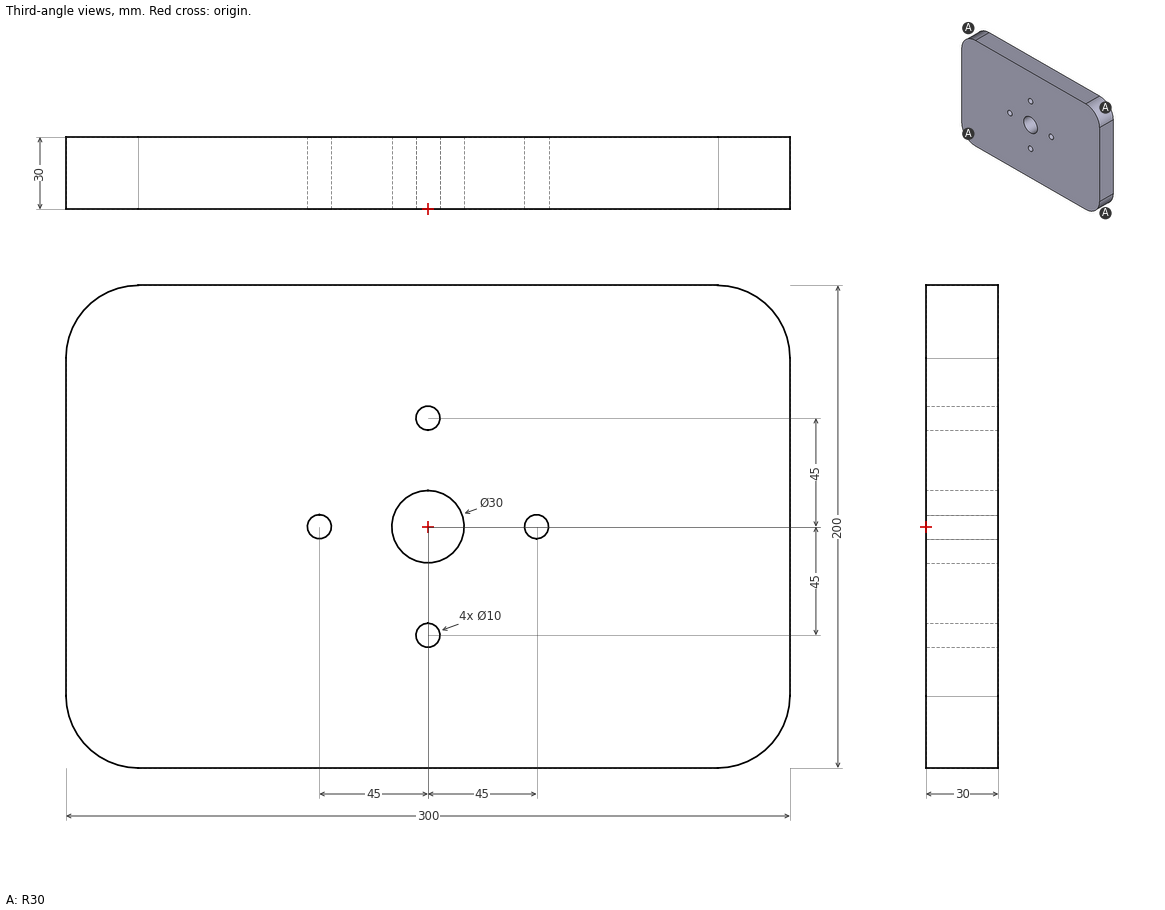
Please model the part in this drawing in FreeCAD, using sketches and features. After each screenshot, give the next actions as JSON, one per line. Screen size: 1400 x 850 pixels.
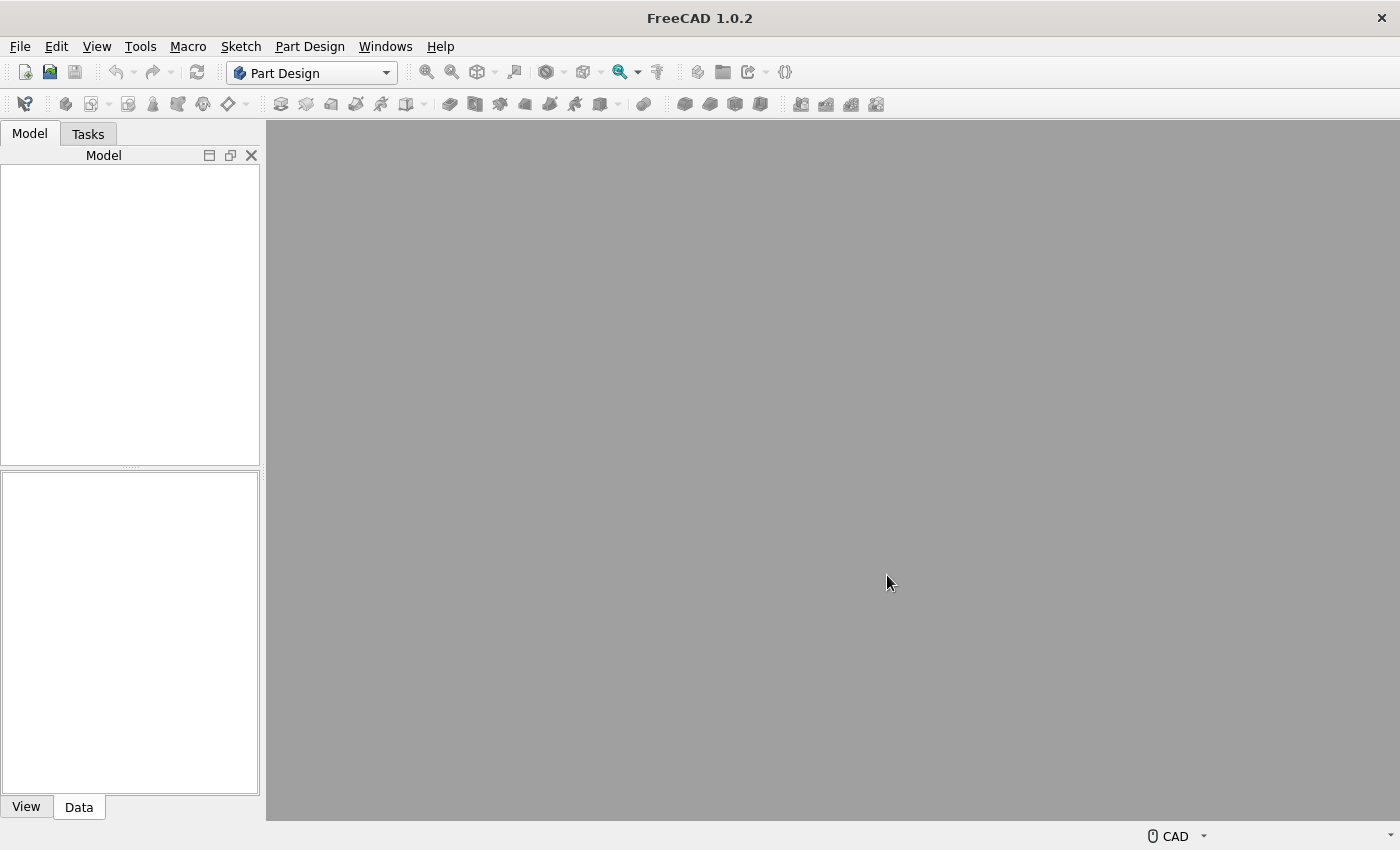
{"action": "key", "text": "ctrl+n"}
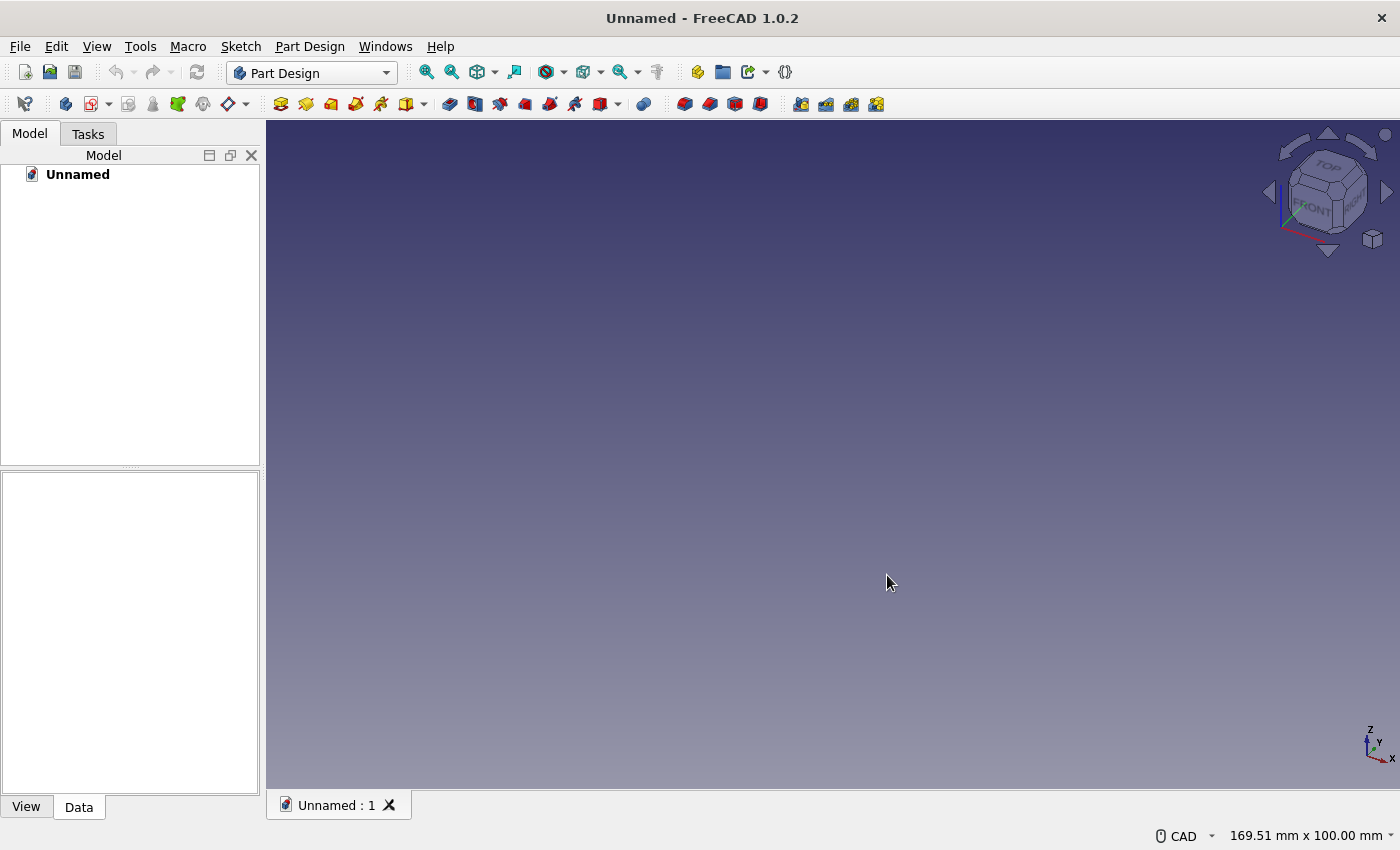
{"action": "left_click", "coordinate": [90, 104]}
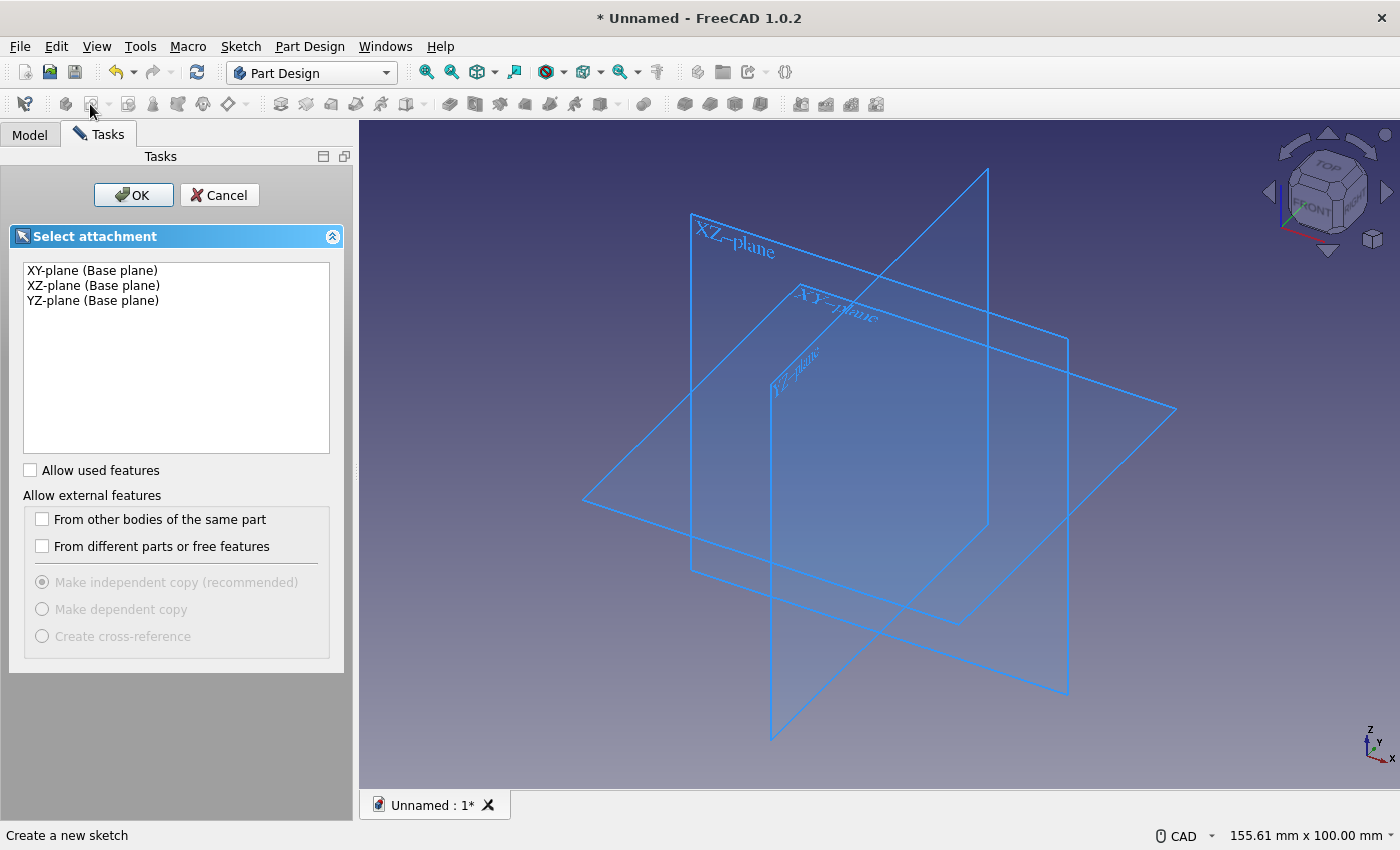
{"action": "left_click", "coordinate": [84, 286]}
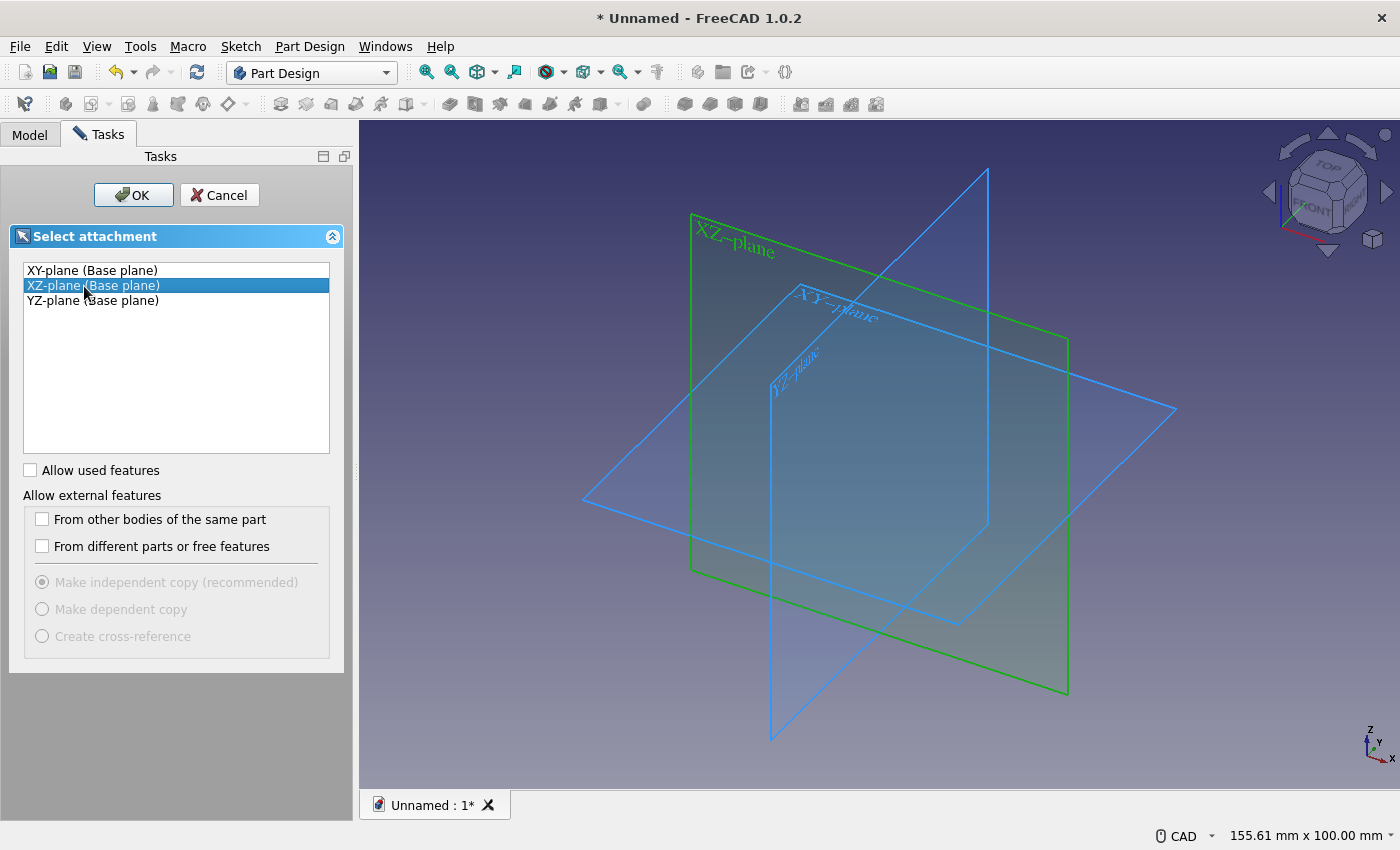
{"action": "left_click", "coordinate": [134, 195]}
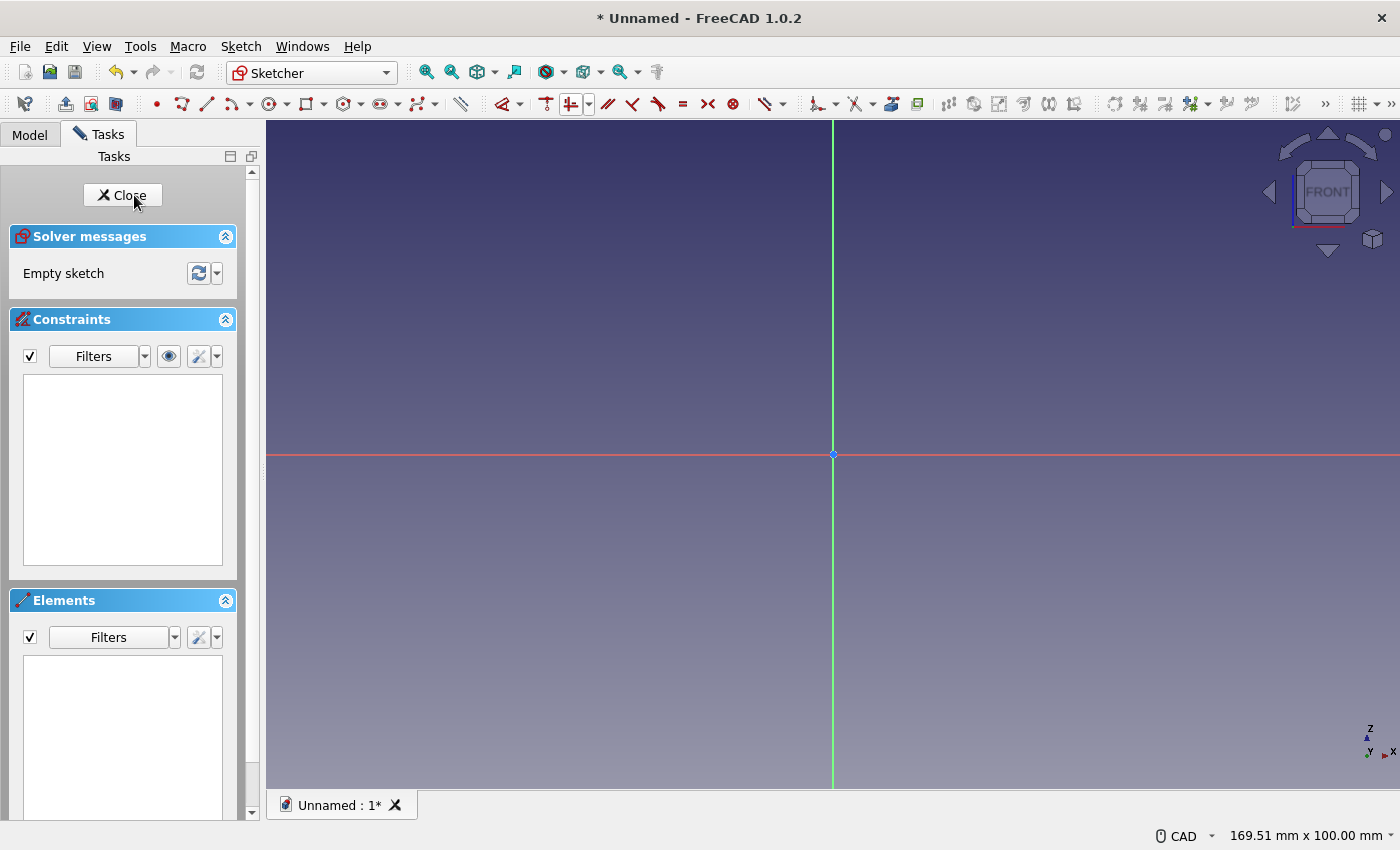
{"action": "scroll", "coordinate": [735, 454], "scroll_direction": "down", "scroll_amount": 6}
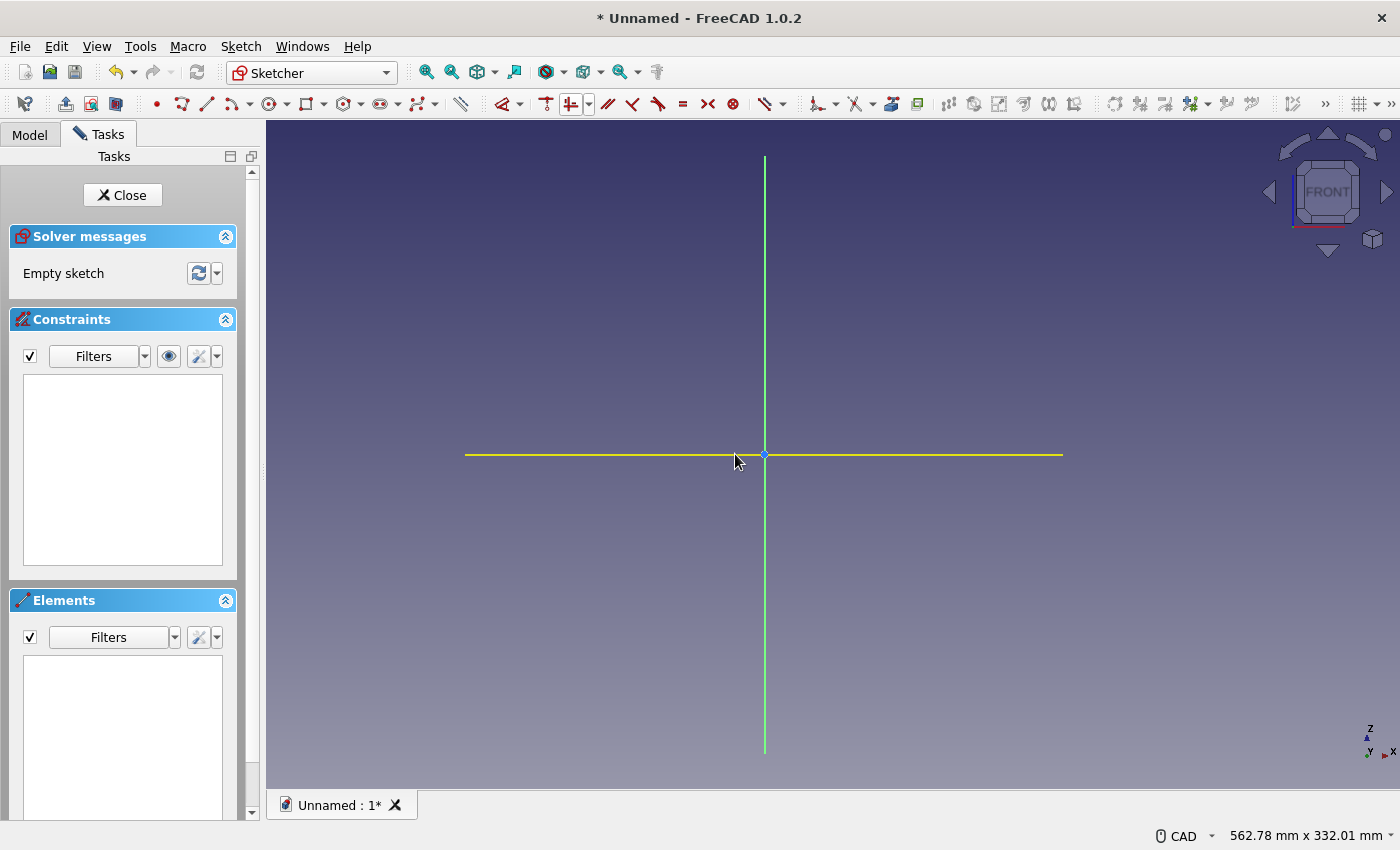
{"action": "key", "text": "g v"}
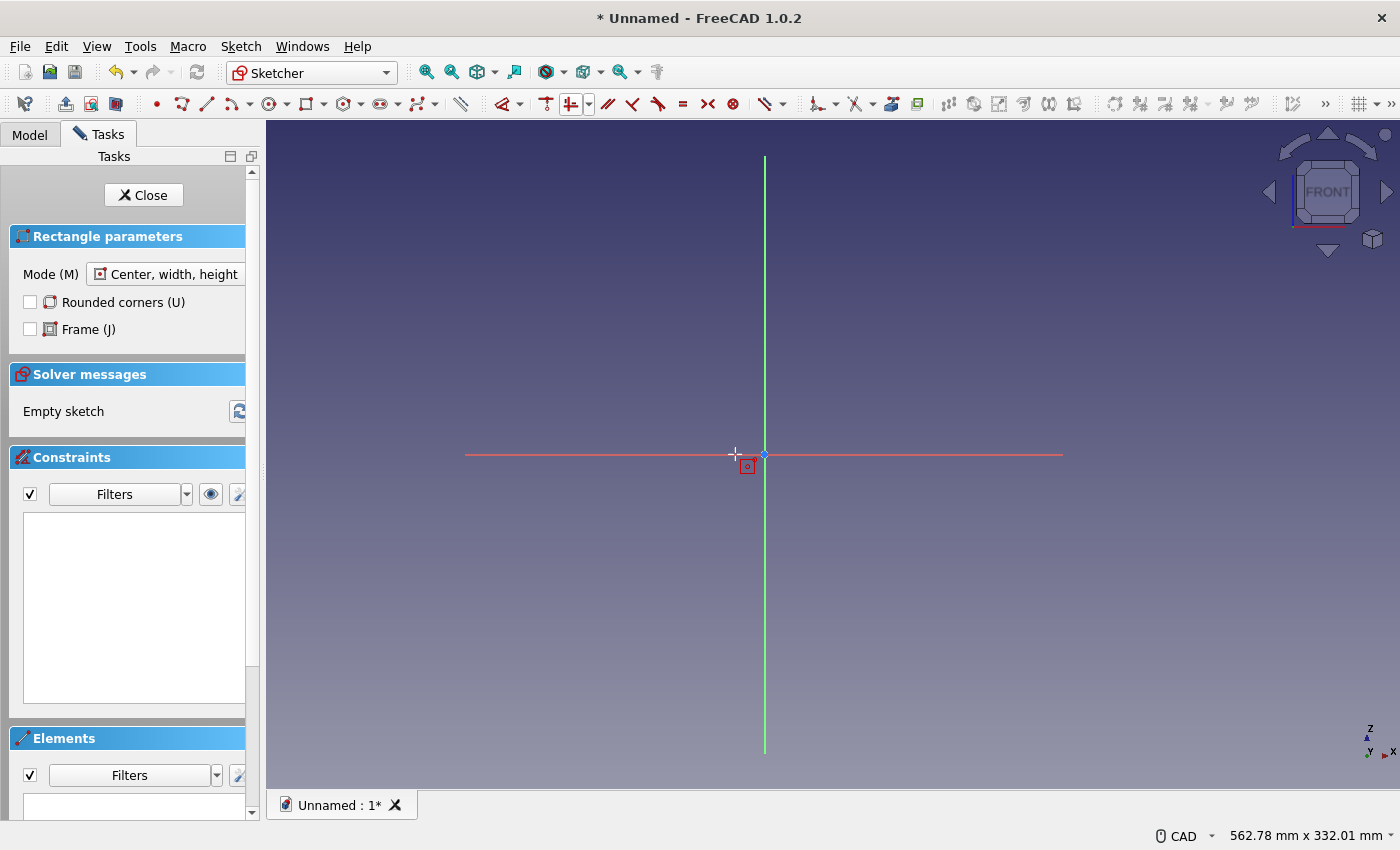
{"action": "left_click", "coordinate": [765, 454]}
{"action": "mouse_move", "coordinate": [1067, 253]}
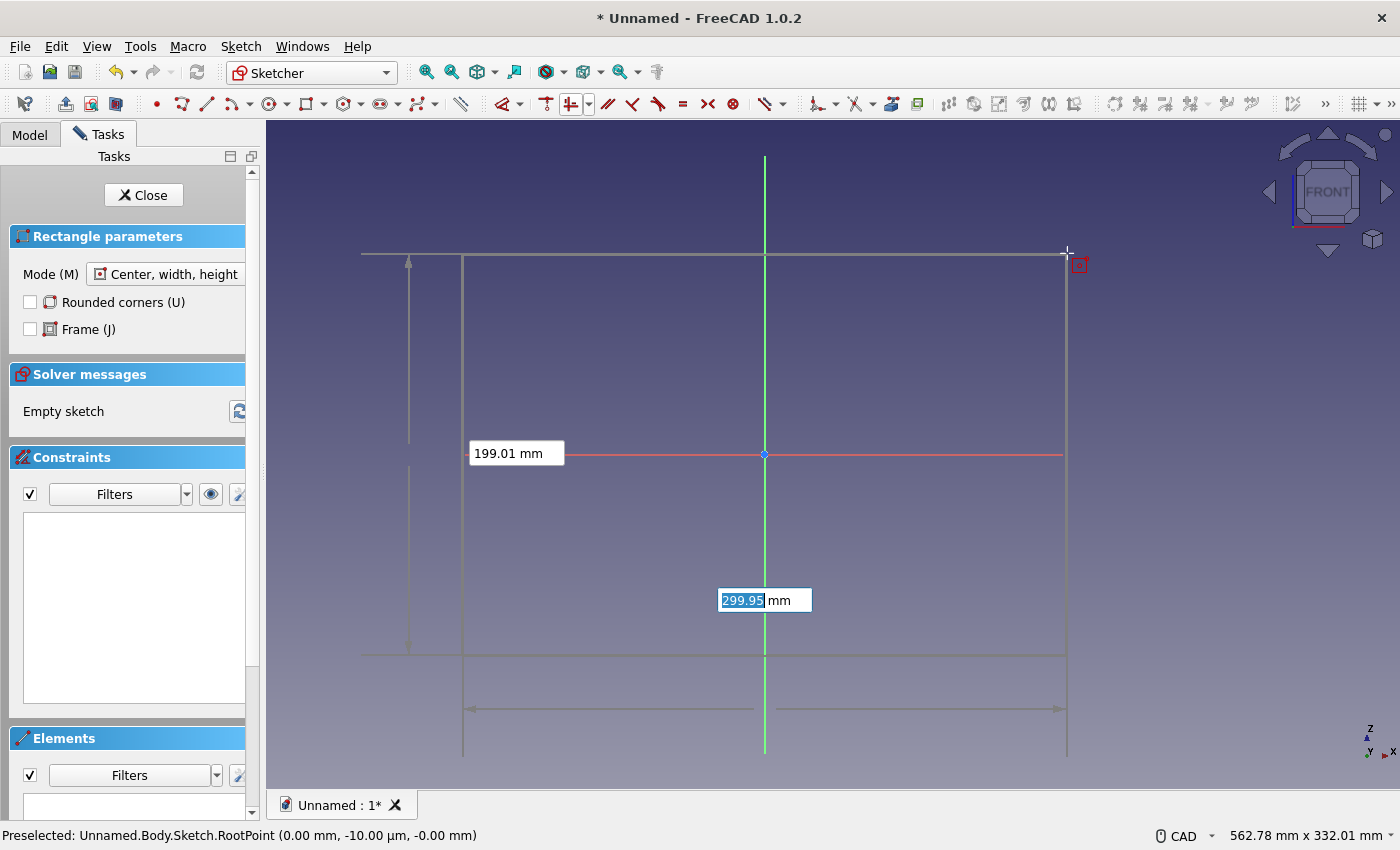
{"action": "type", "text": "300"}
{"action": "key", "text": "Tab"}
{"action": "type", "text": "200"}
{"action": "key", "text": "Return"}
{"action": "key", "text": "Escape"}